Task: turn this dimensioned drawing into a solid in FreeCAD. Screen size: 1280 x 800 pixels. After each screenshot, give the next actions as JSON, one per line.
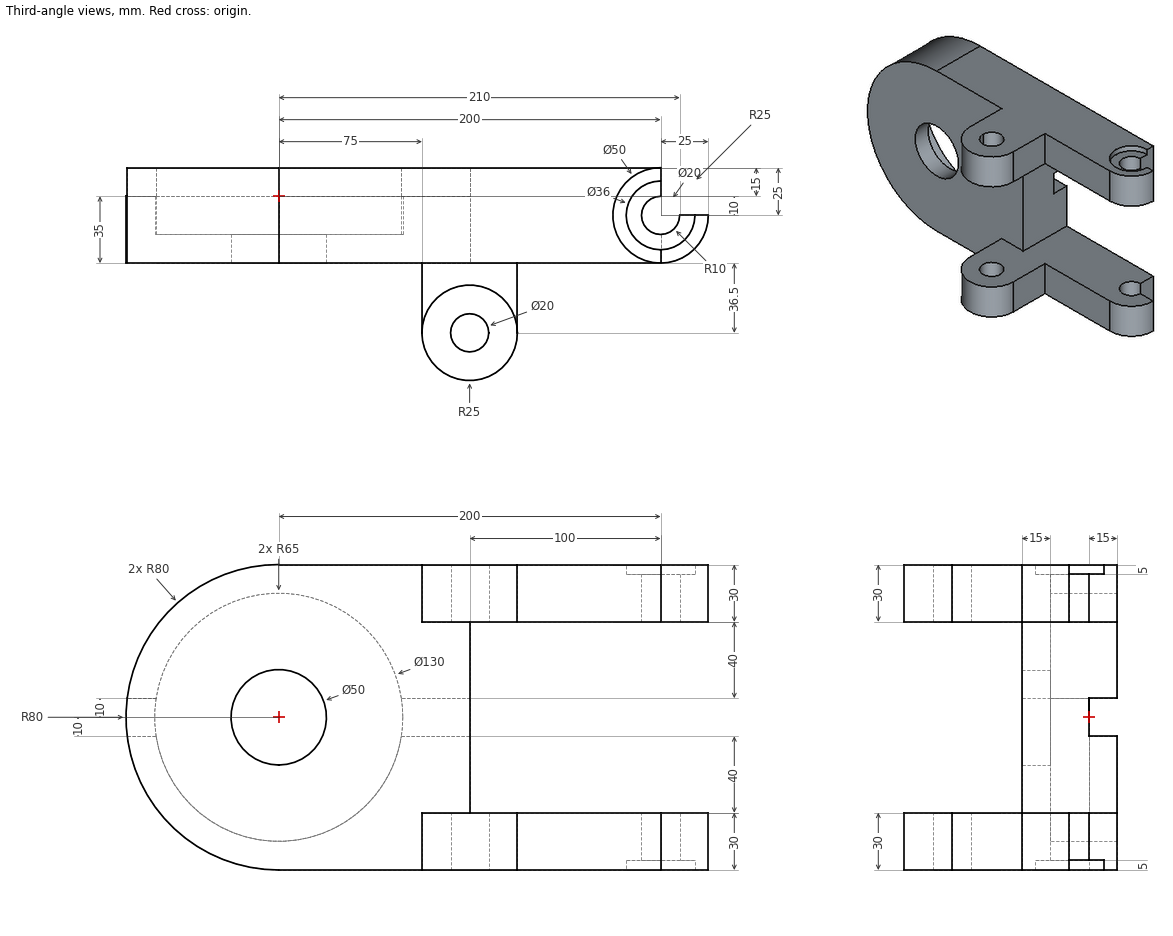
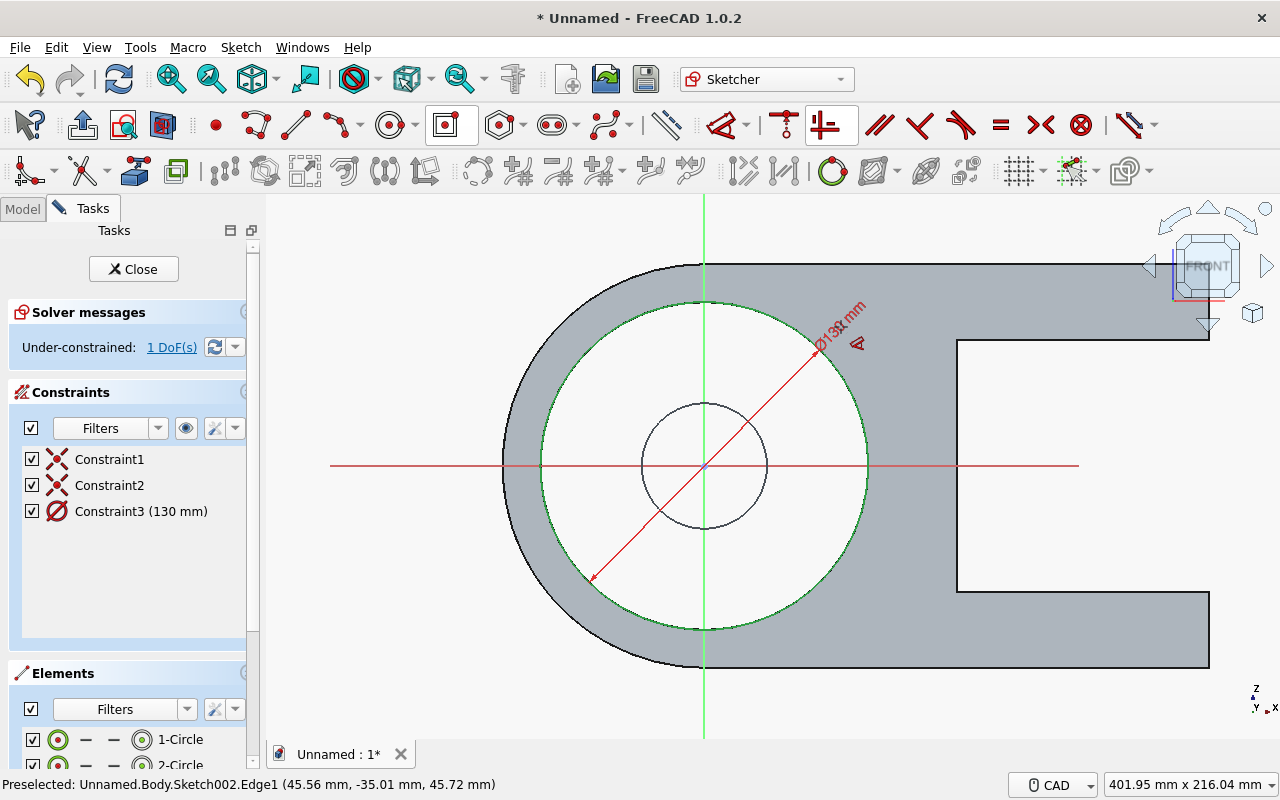
{"action": "left_click", "coordinate": [749, 422]}
{"action": "left_click", "coordinate": [772, 400]}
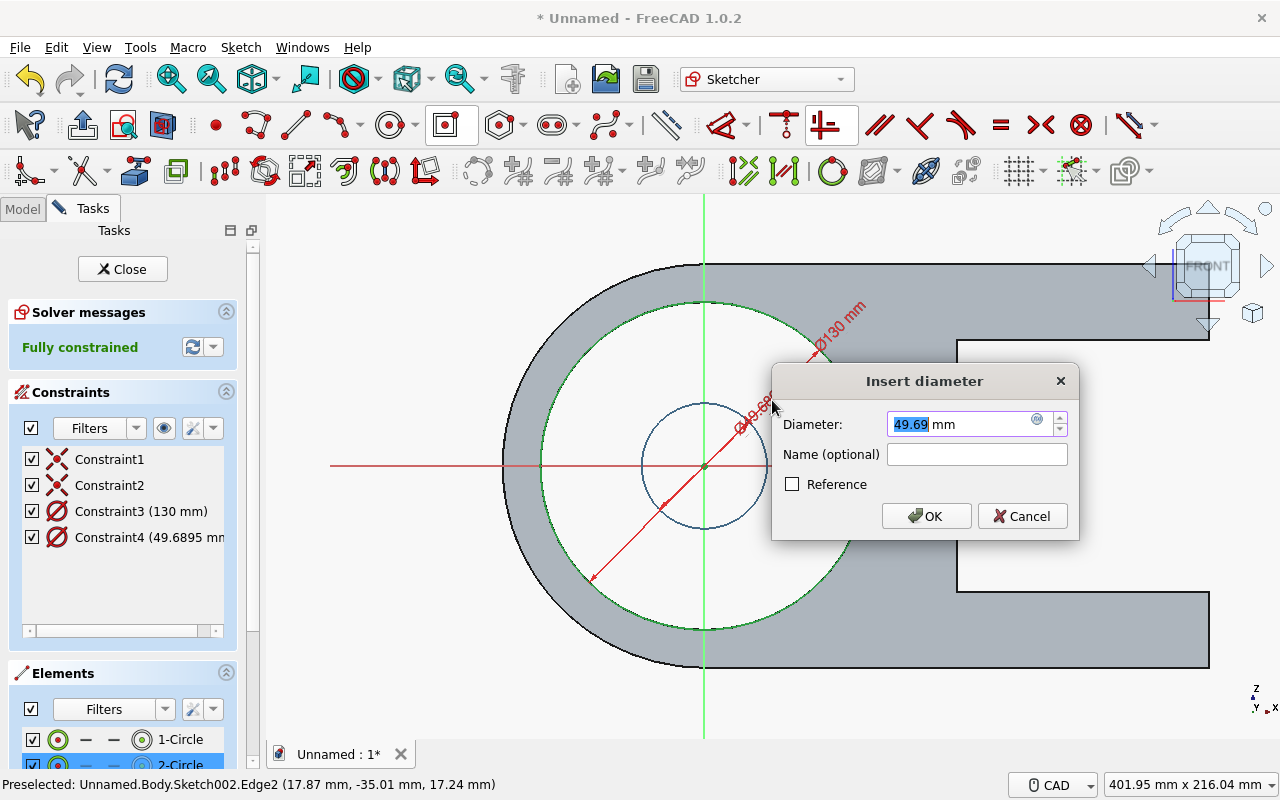
{"action": "type", "text": "50"}
{"action": "key", "text": "Return"}
{"action": "key", "text": "Escape"}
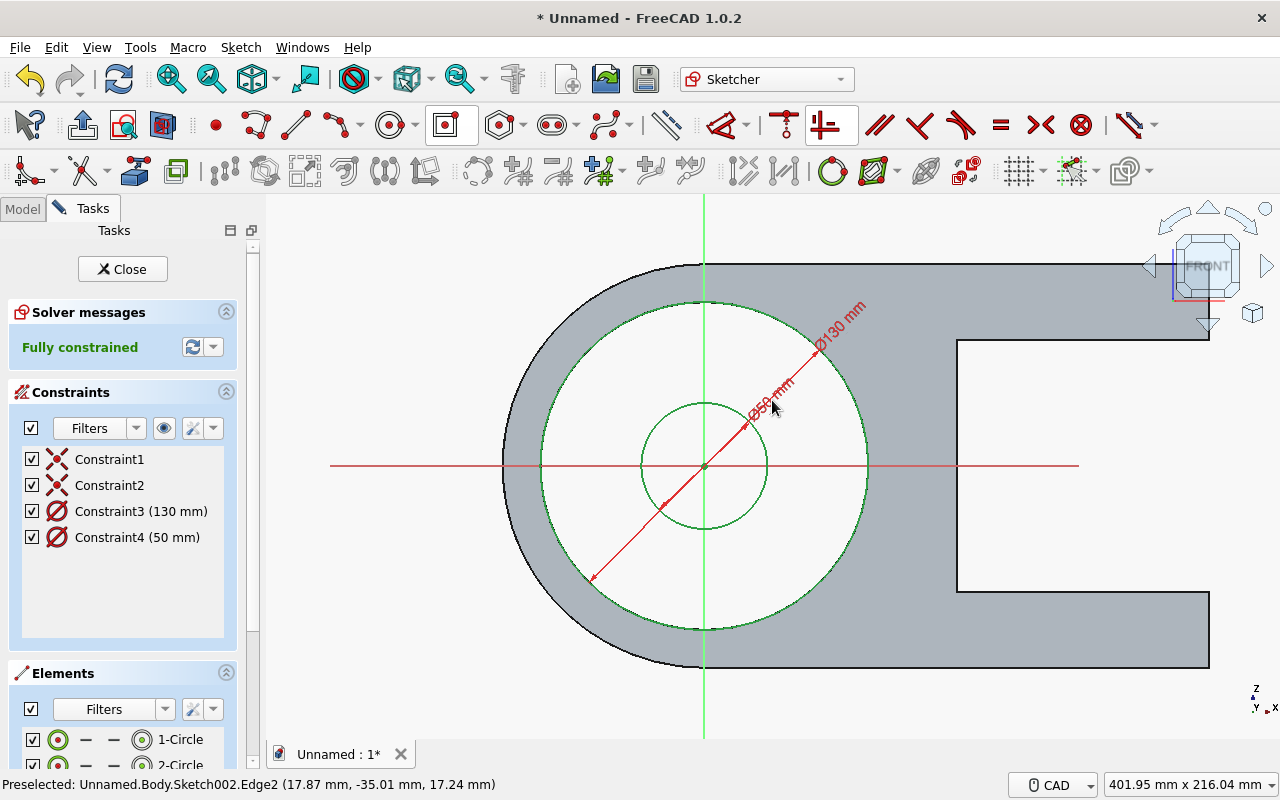
{"action": "left_click", "coordinate": [123, 269]}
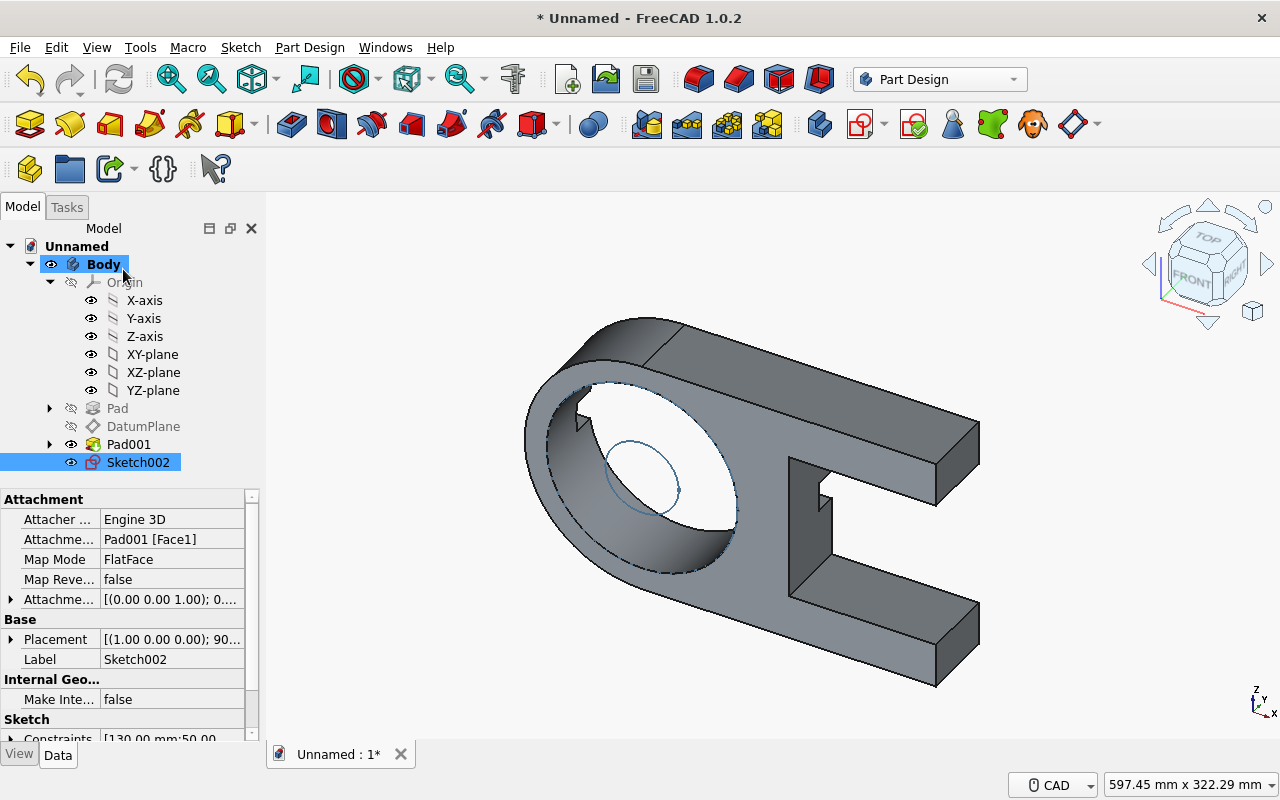
{"action": "left_click", "coordinate": [30, 124]}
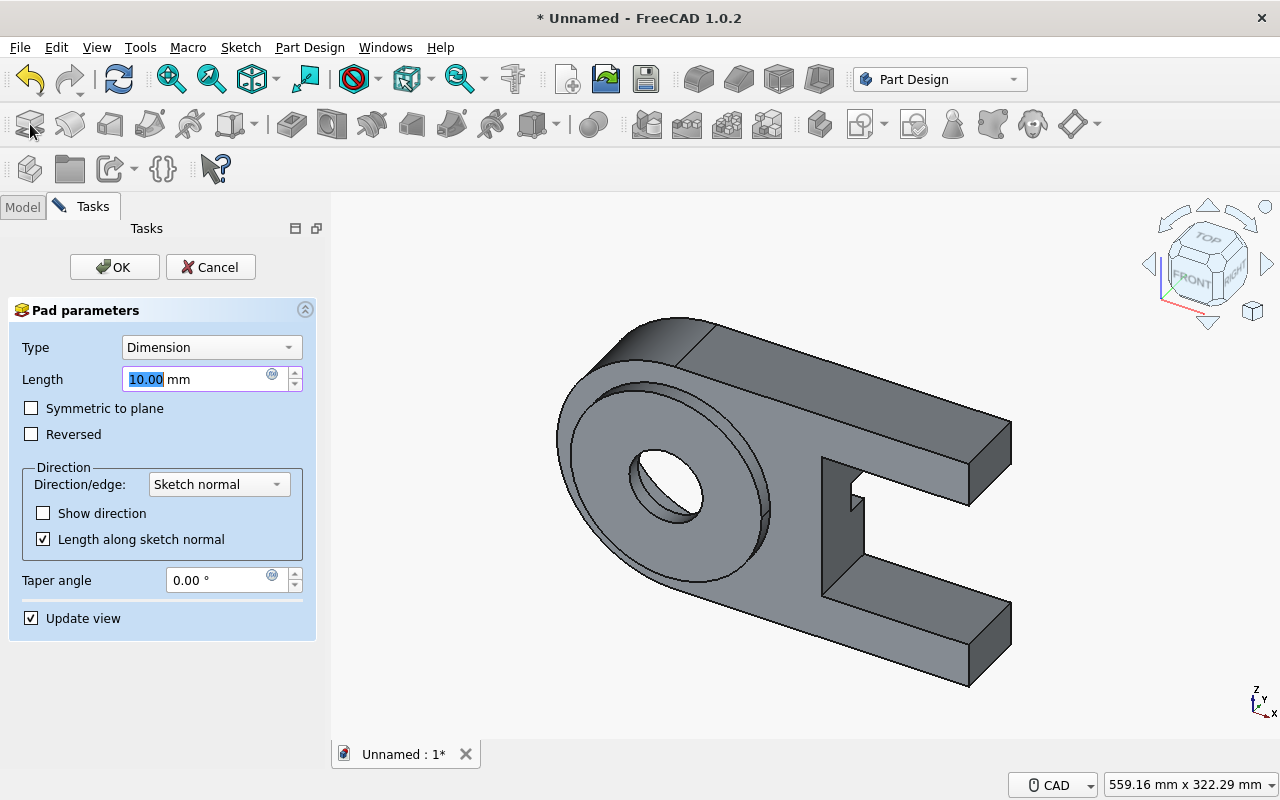
{"action": "type", "text": "15"}
{"action": "key", "text": "Tab"}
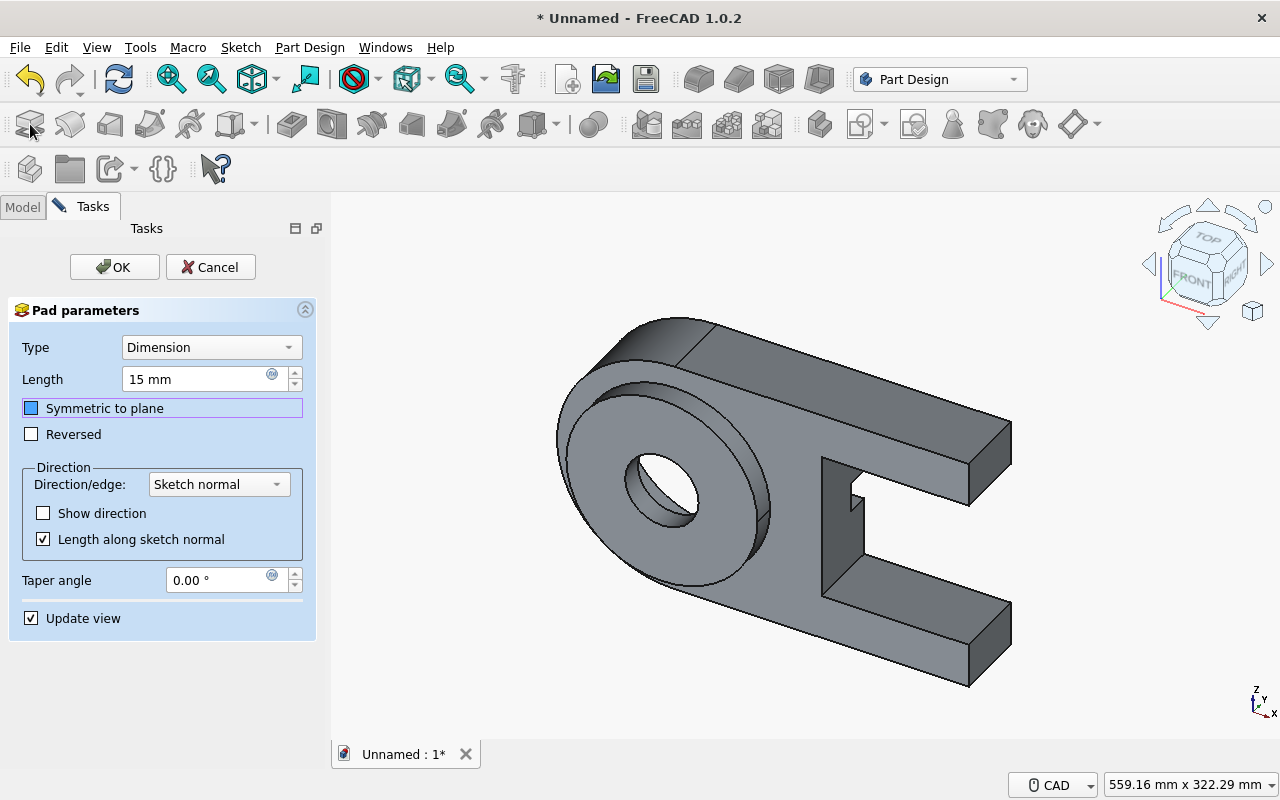
{"action": "left_click", "coordinate": [30, 434]}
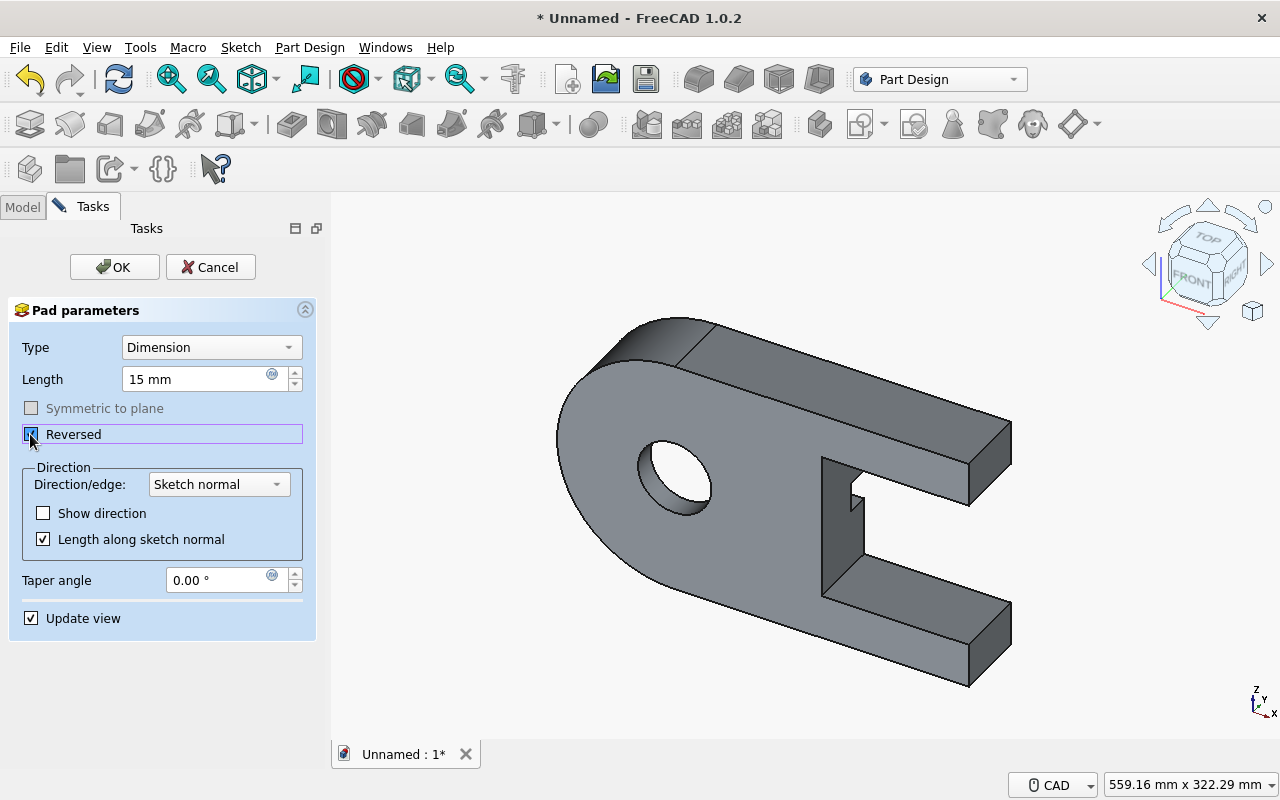
{"action": "left_click", "coordinate": [115, 267]}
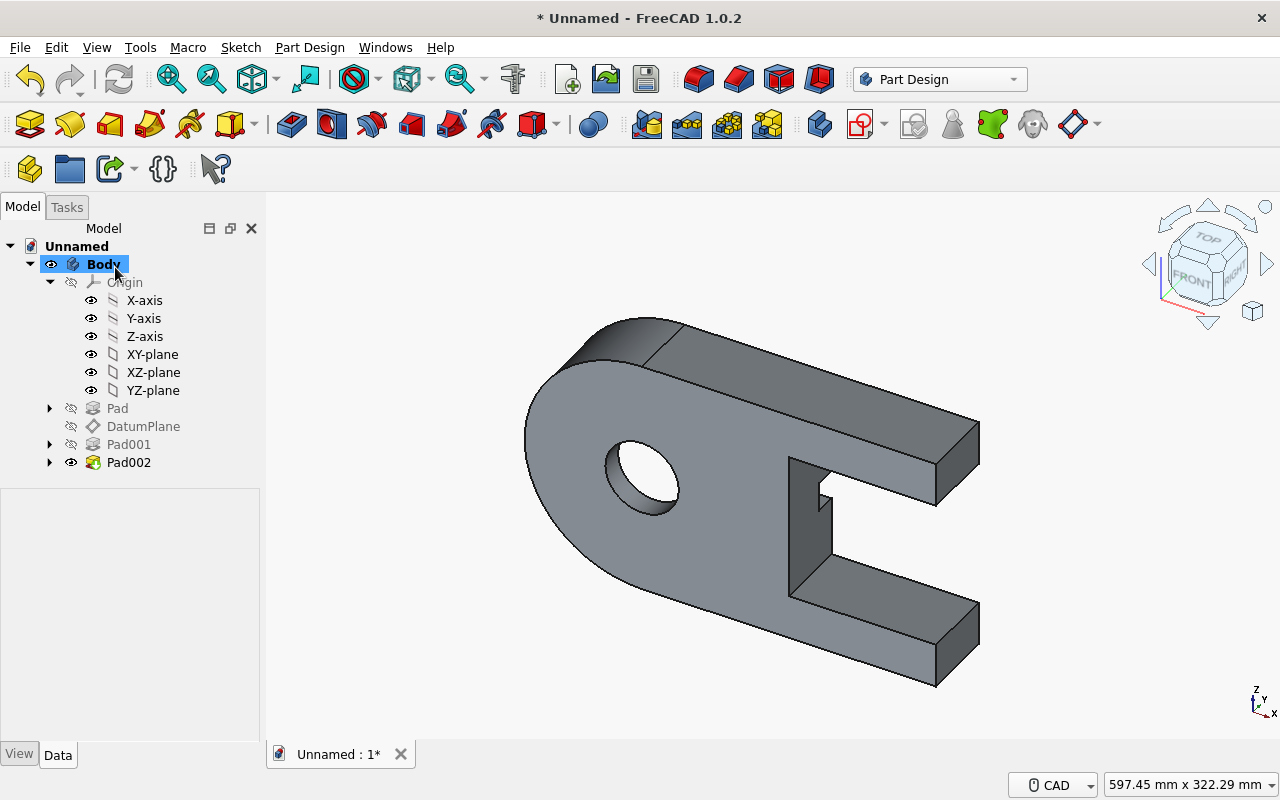
{"action": "left_click", "coordinate": [894, 421]}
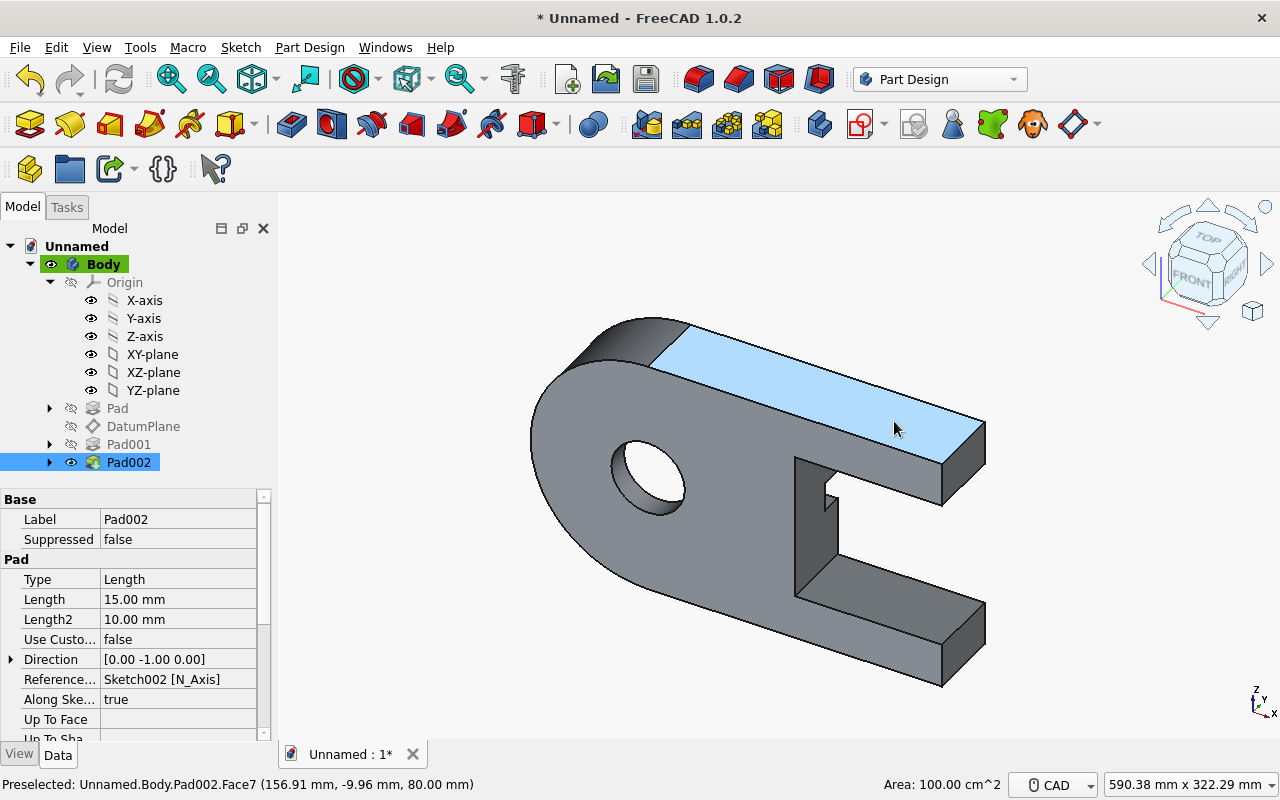
{"action": "left_click", "coordinate": [860, 124]}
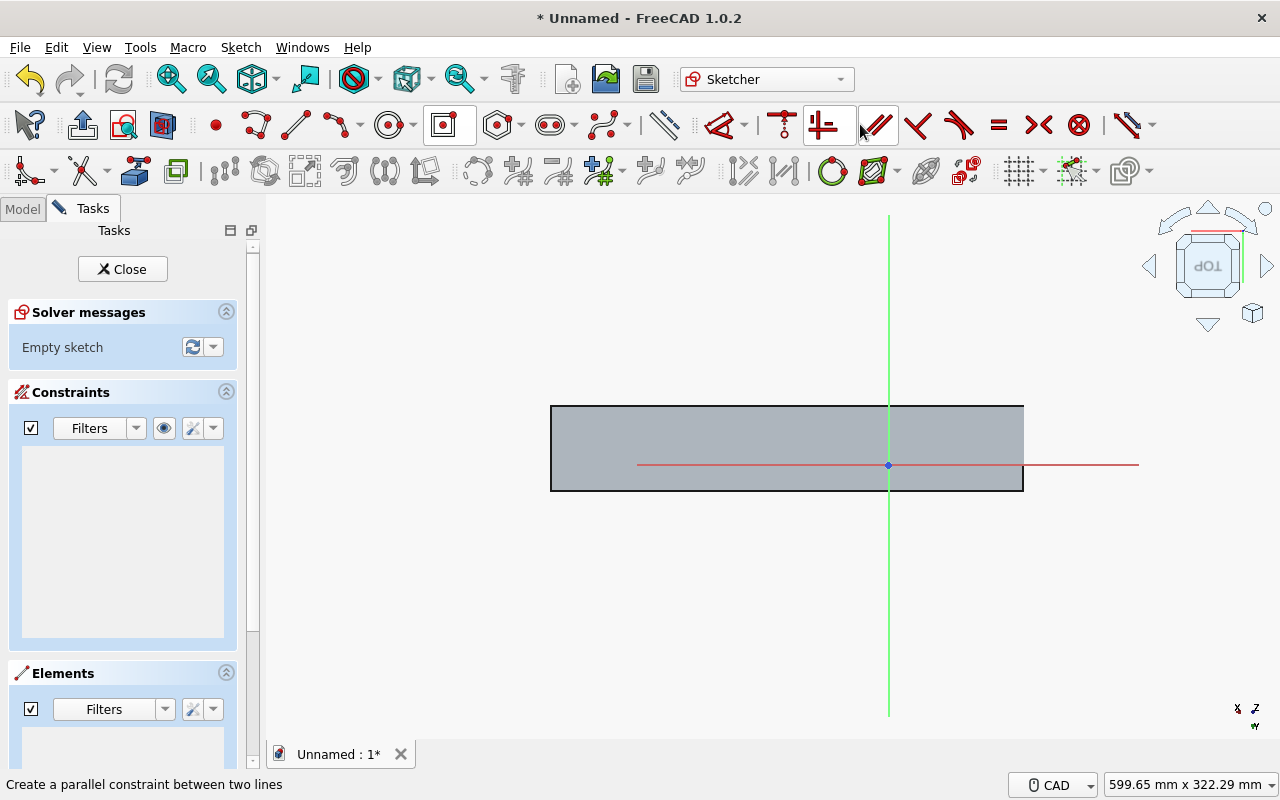
{"action": "scroll", "coordinate": [847, 316], "scroll_direction": "up", "scroll_amount": 4}